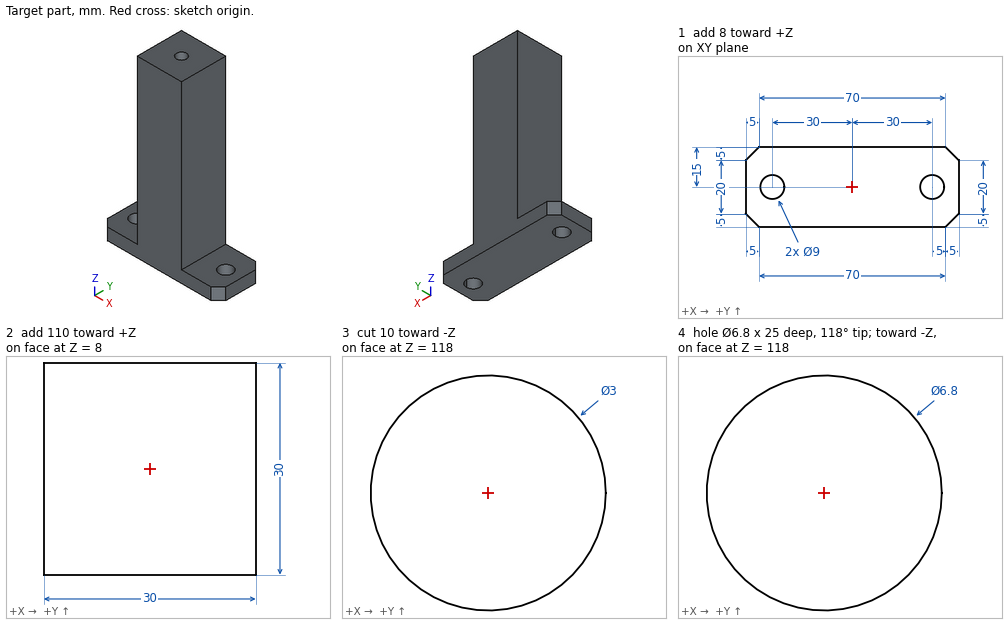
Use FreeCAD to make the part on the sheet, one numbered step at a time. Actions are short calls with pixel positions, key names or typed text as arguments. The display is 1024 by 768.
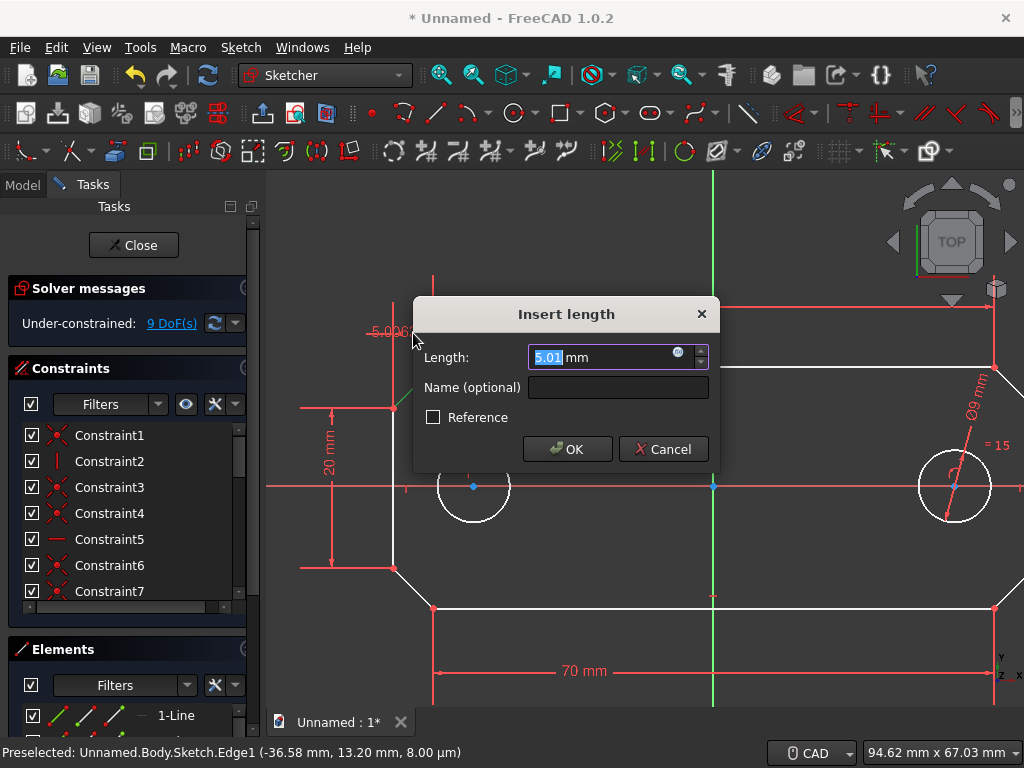
text(5)
key(Return)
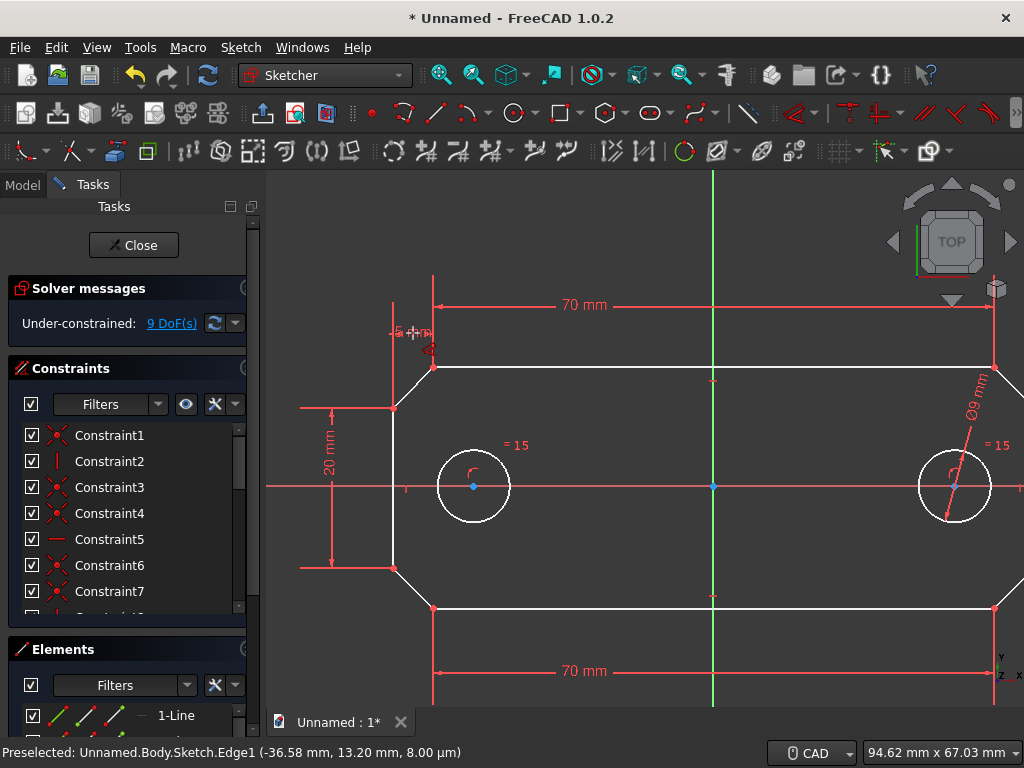
click(421, 380)
click(359, 388)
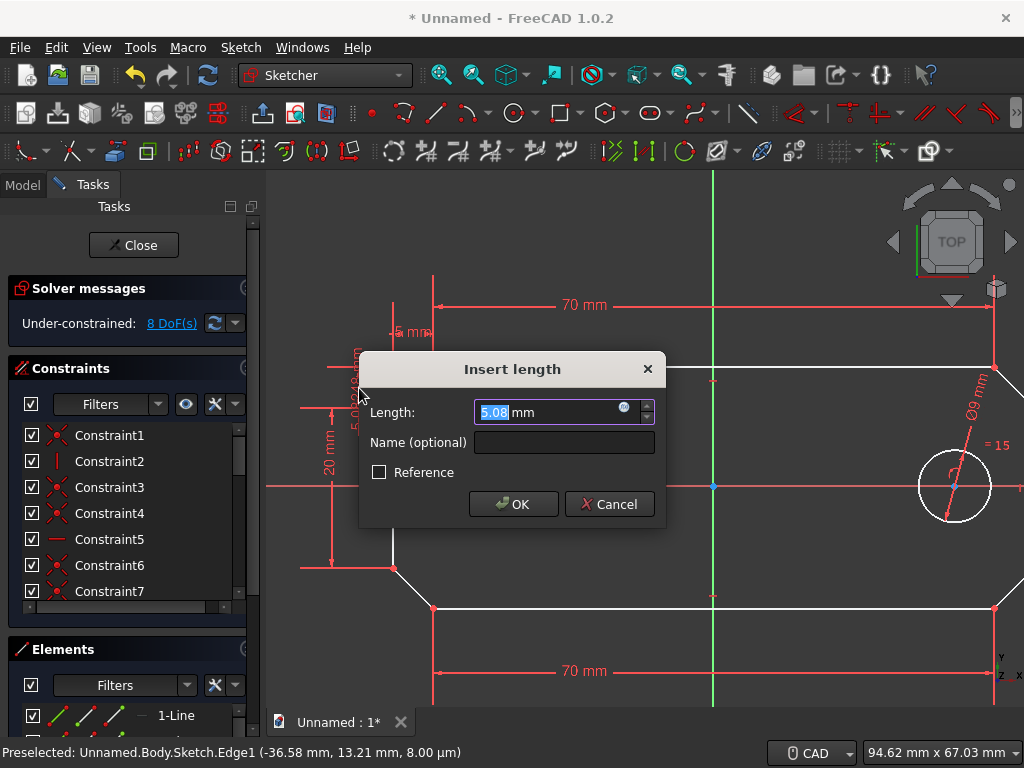
text(5)
key(Return)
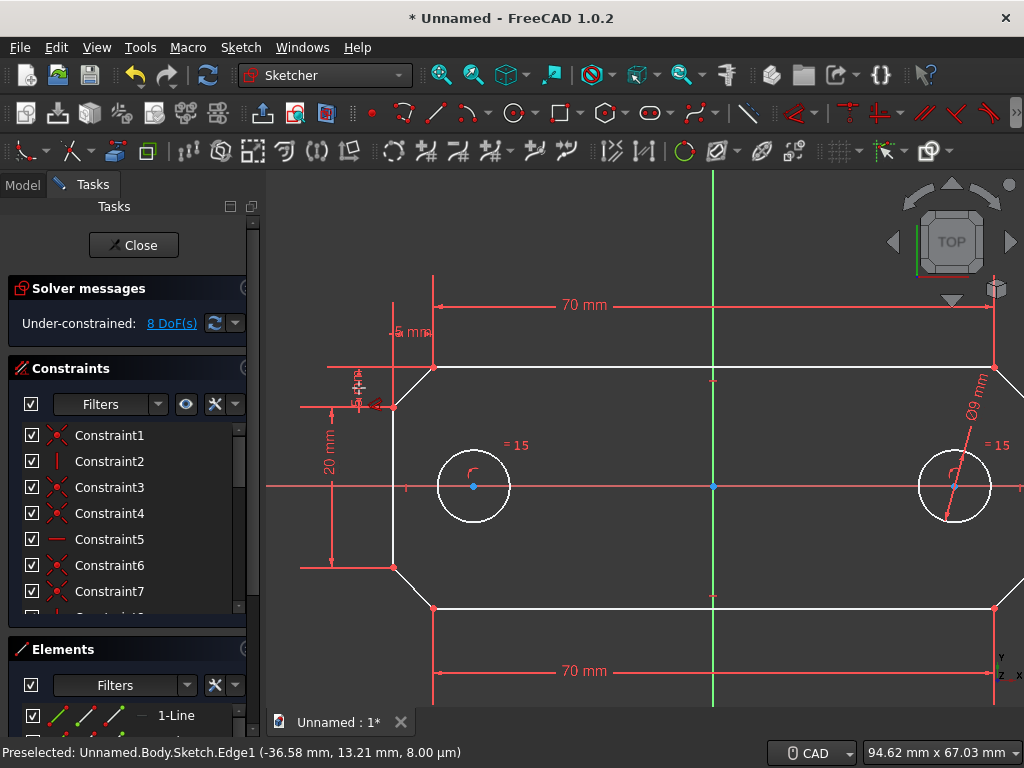
click(405, 580)
click(413, 643)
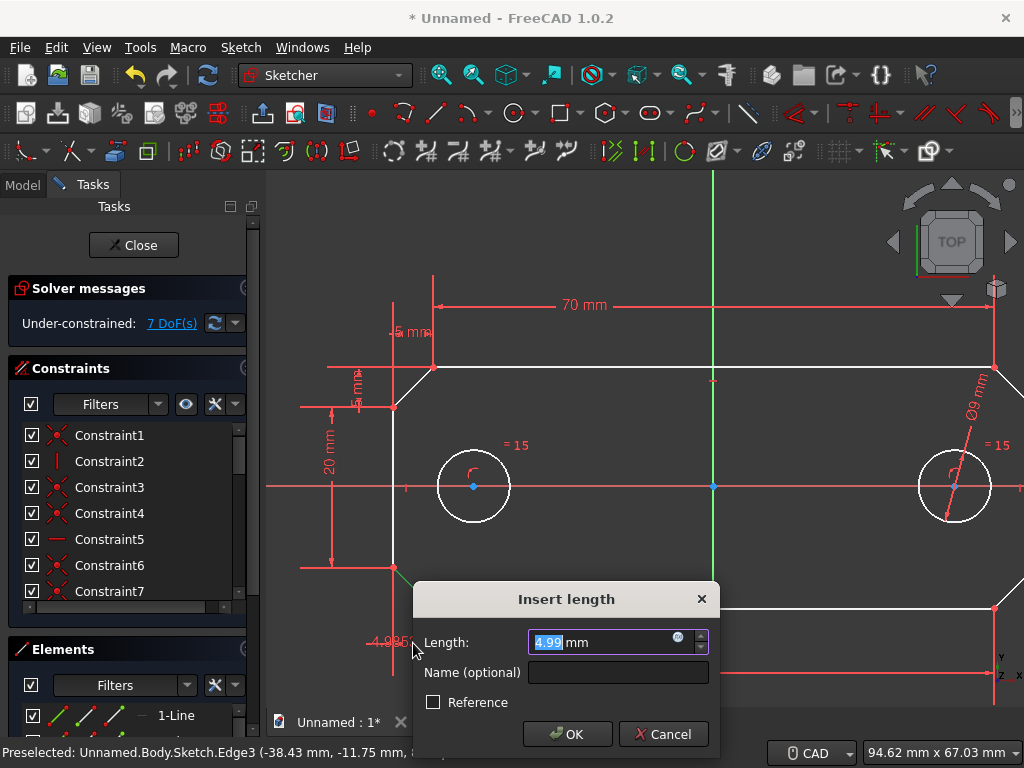
text(5)
key(Return)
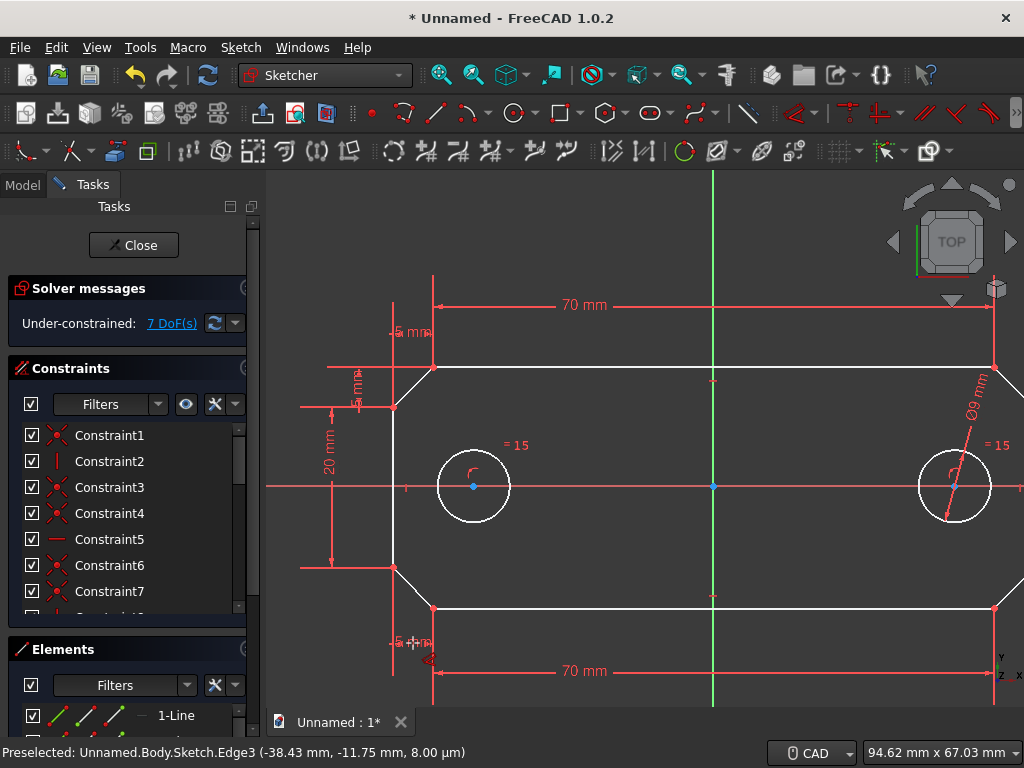
click(405, 580)
click(359, 588)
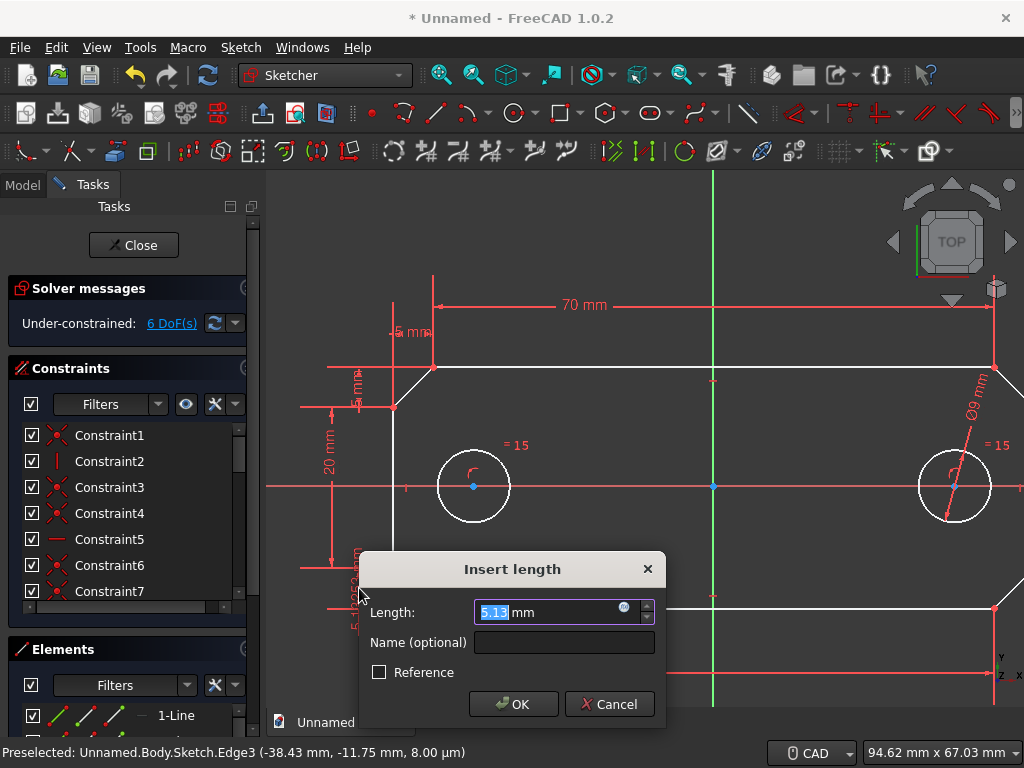
text(5)
key(Return)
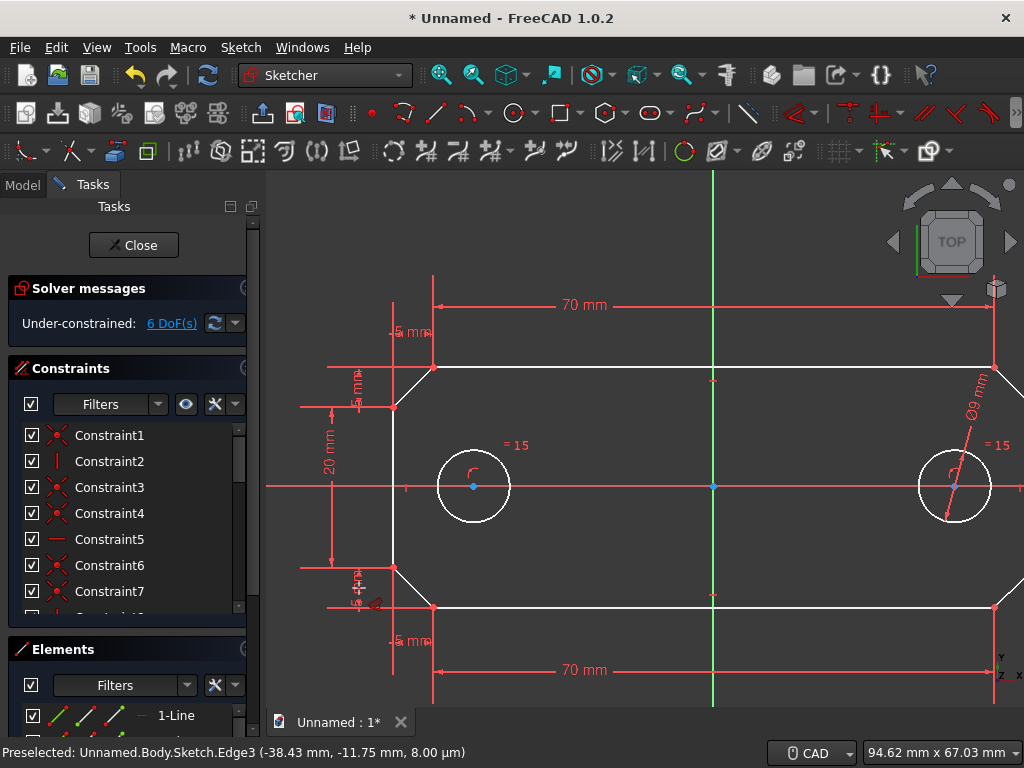
scroll(298, 341, down, 2)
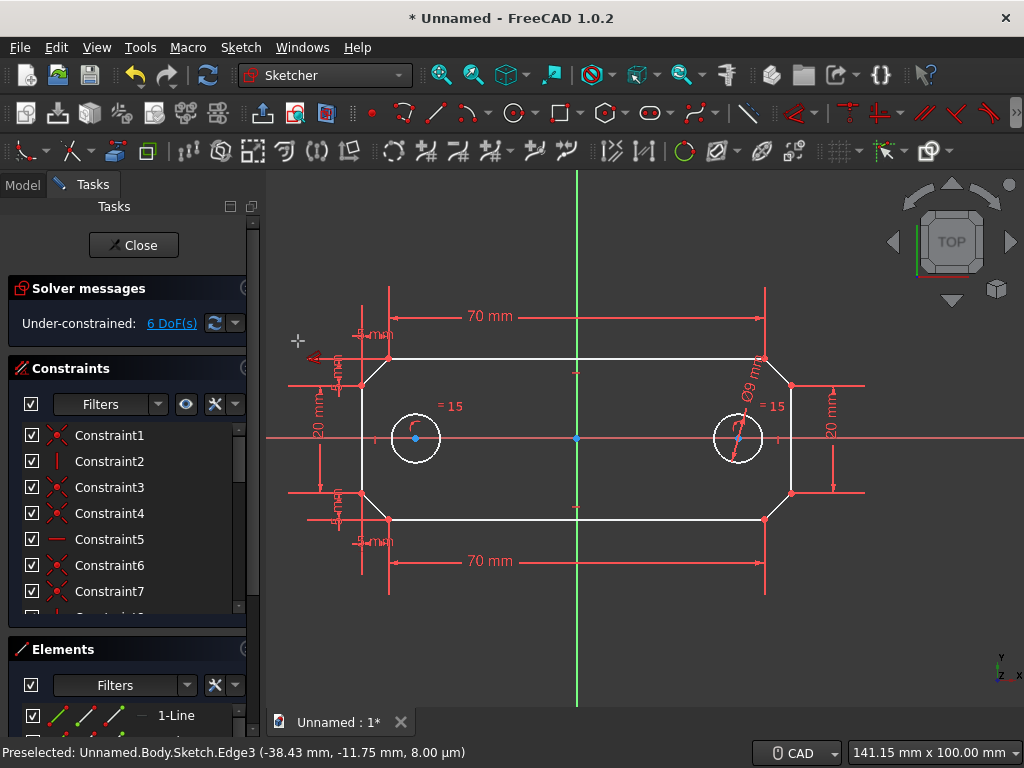
scroll(773, 512, up, 2)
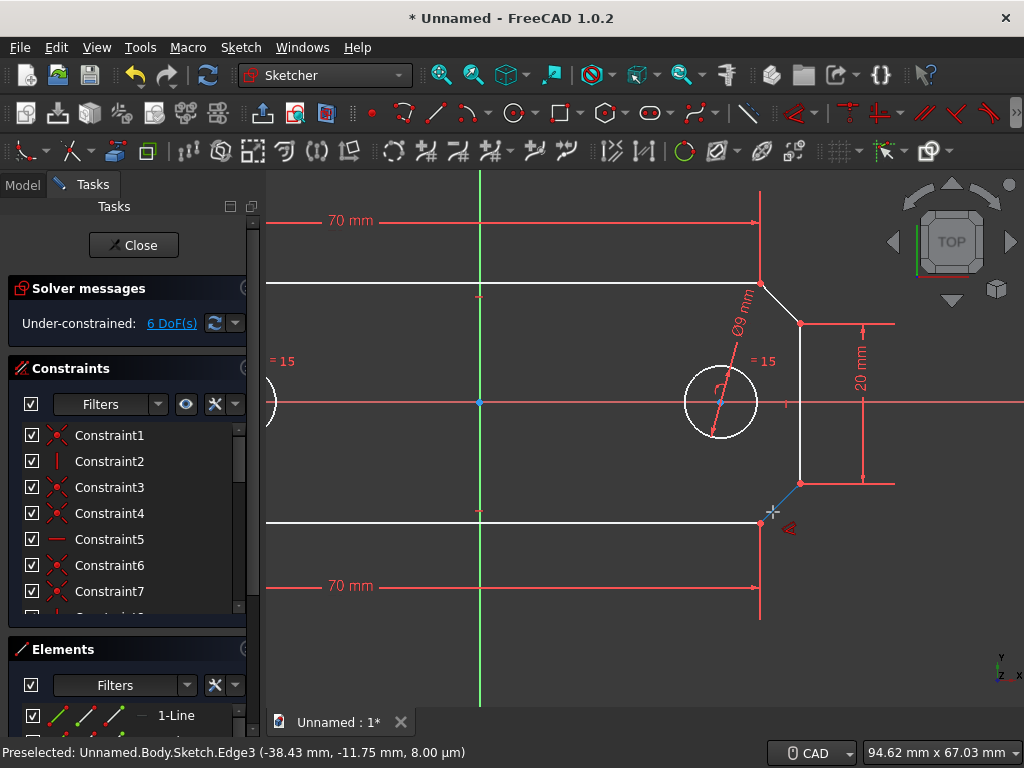
click(772, 512)
click(780, 557)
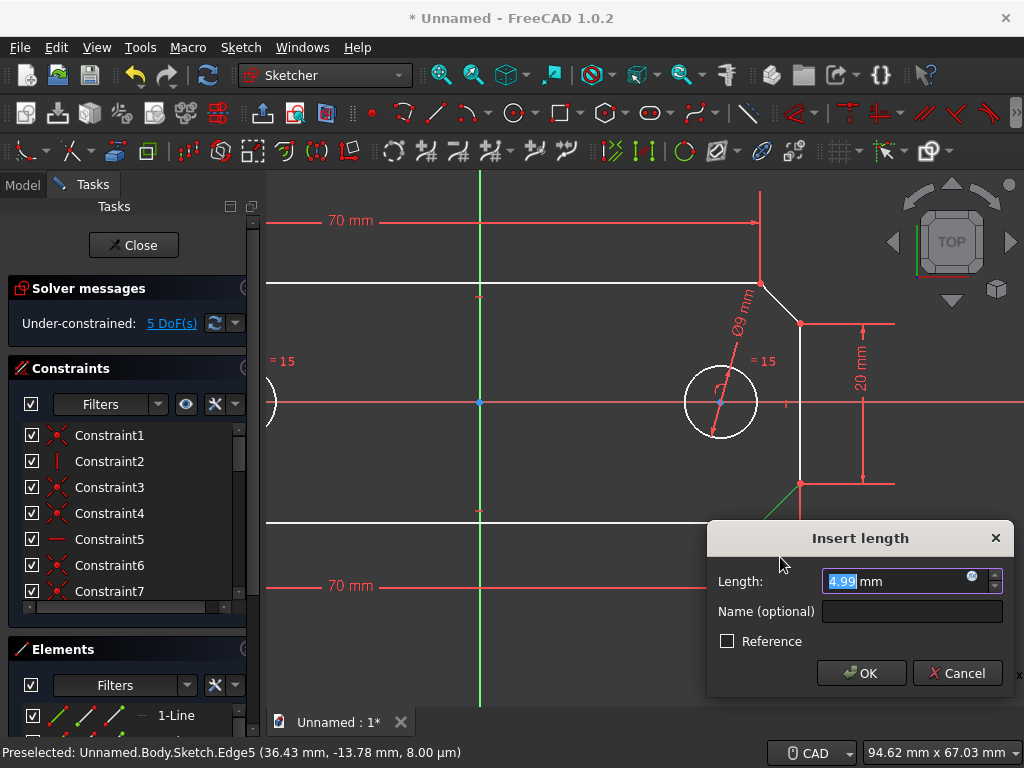
text(5)
key(Return)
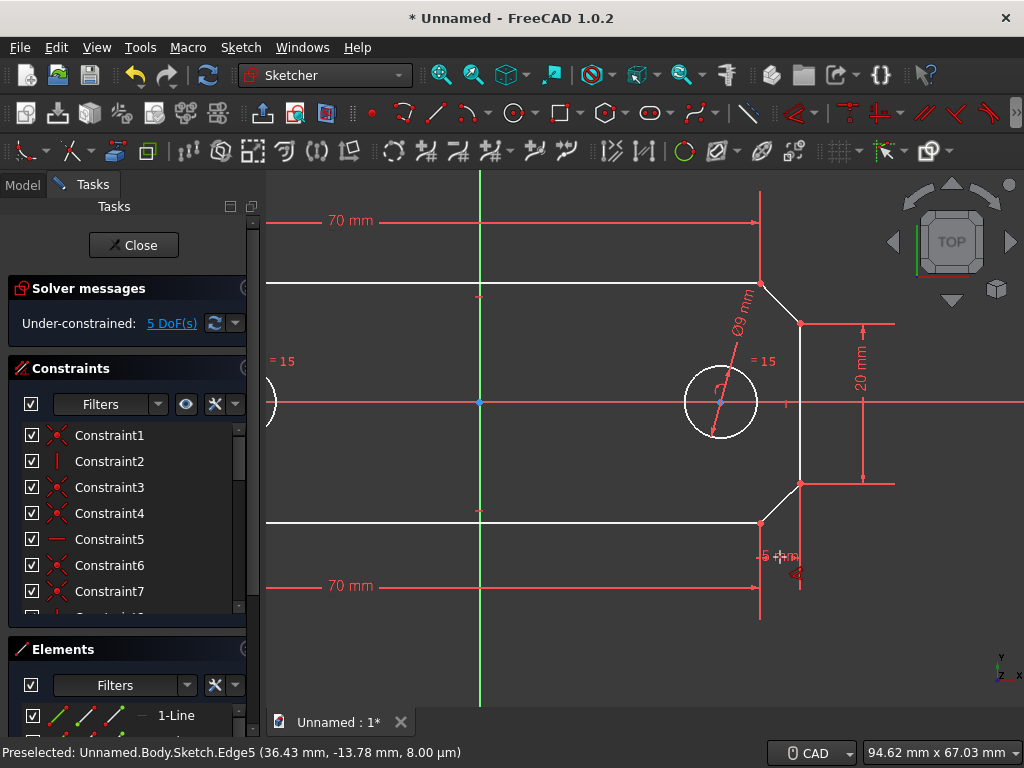
click(772, 512)
click(834, 504)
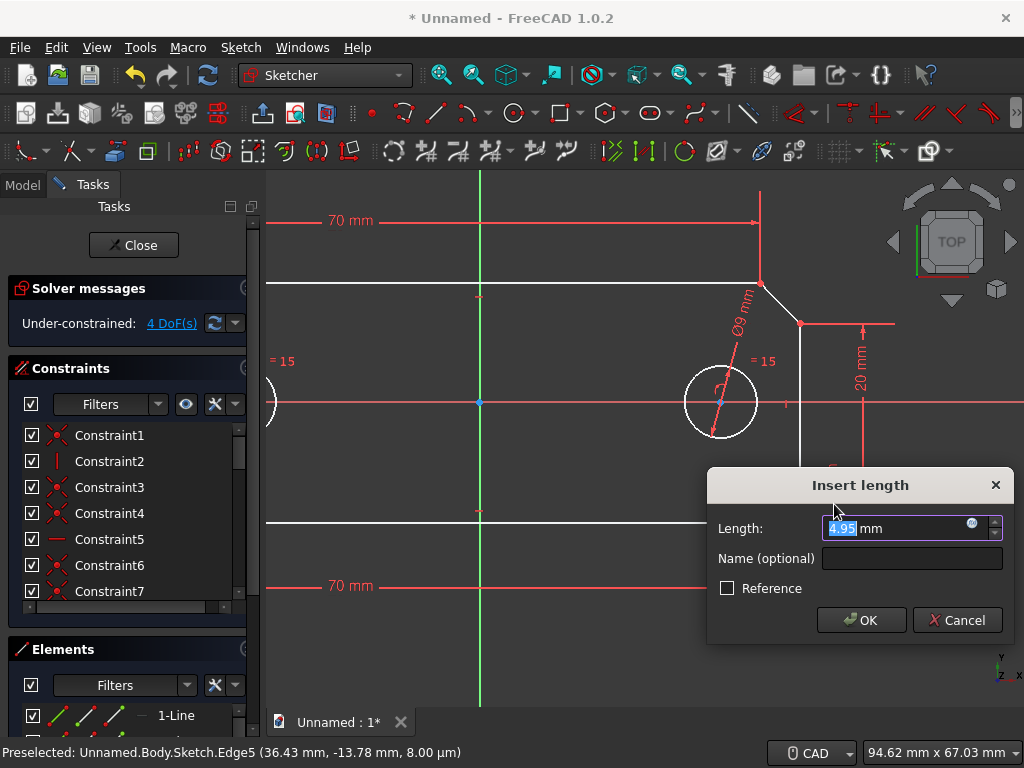
text(5)
key(Return)